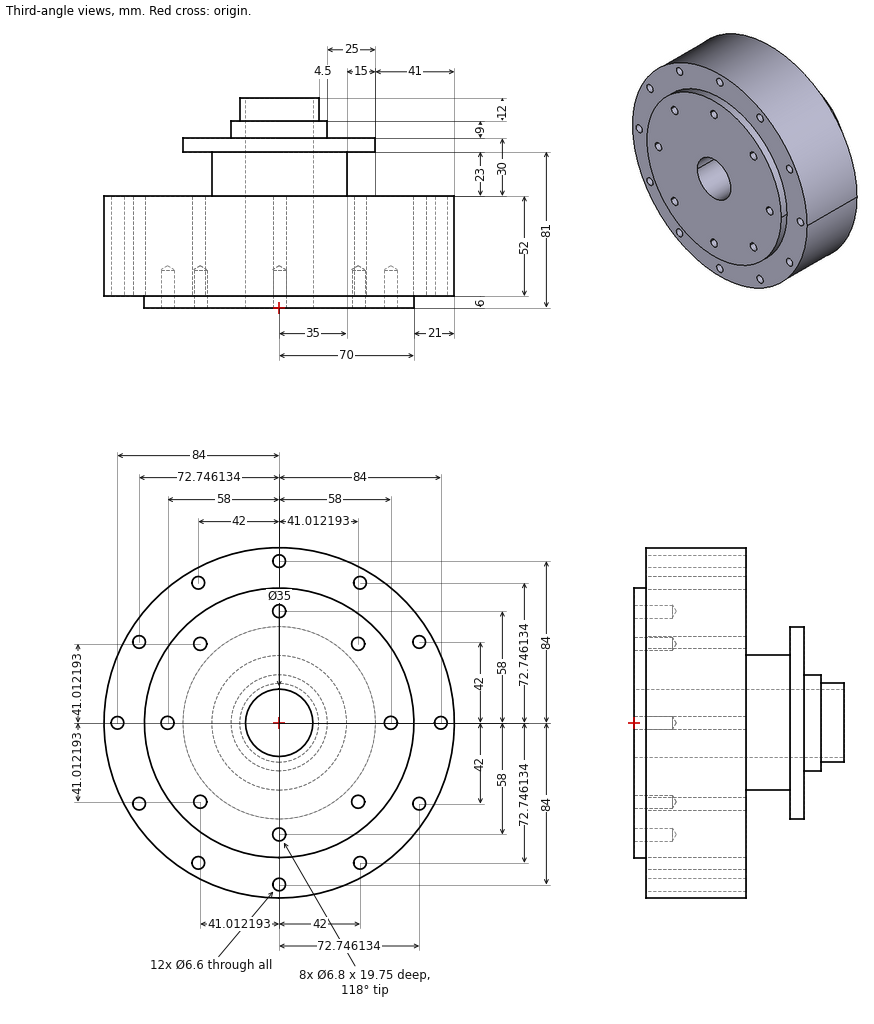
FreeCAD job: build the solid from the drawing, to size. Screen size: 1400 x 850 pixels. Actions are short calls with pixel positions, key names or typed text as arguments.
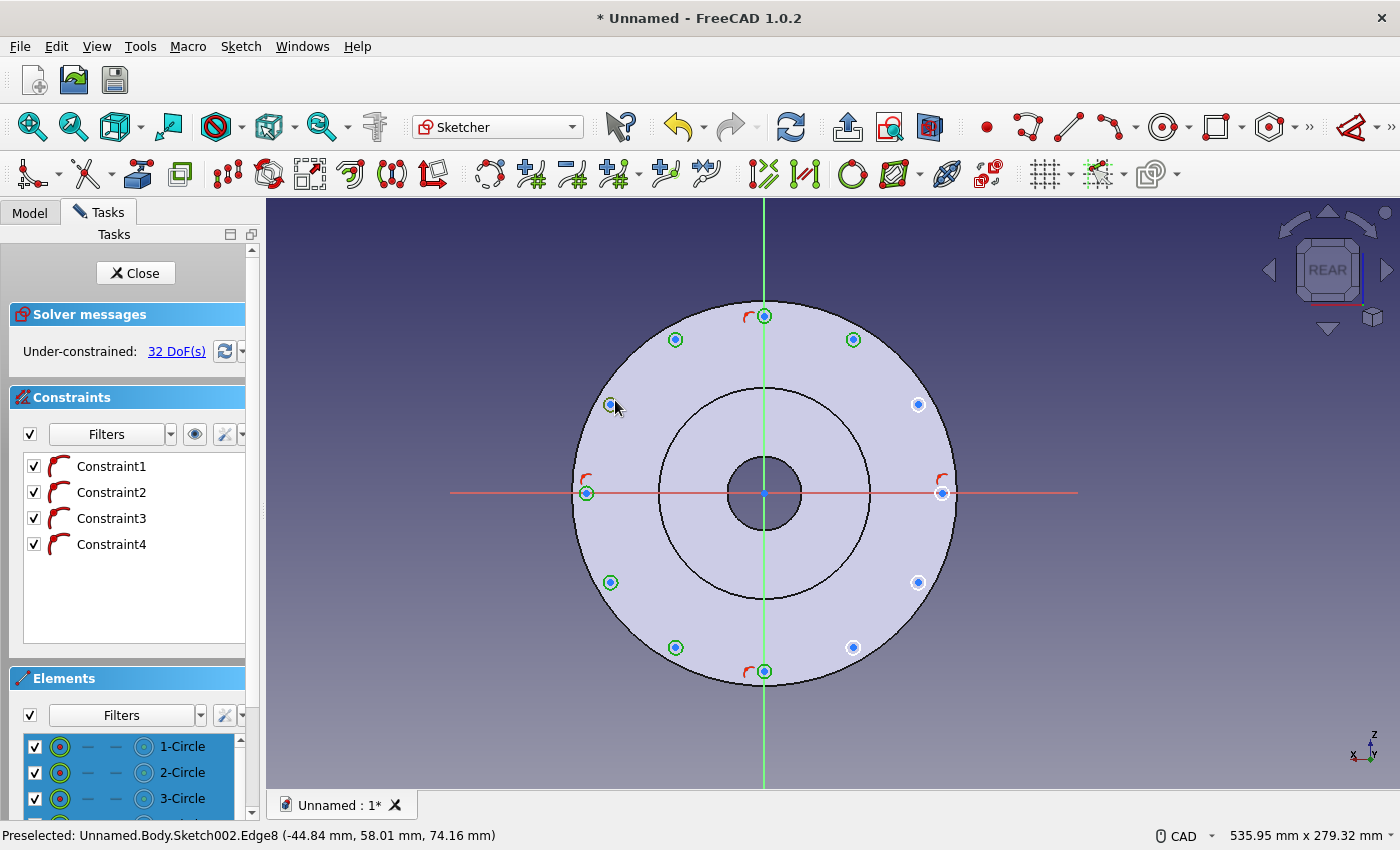
scroll(923, 400, up, 4)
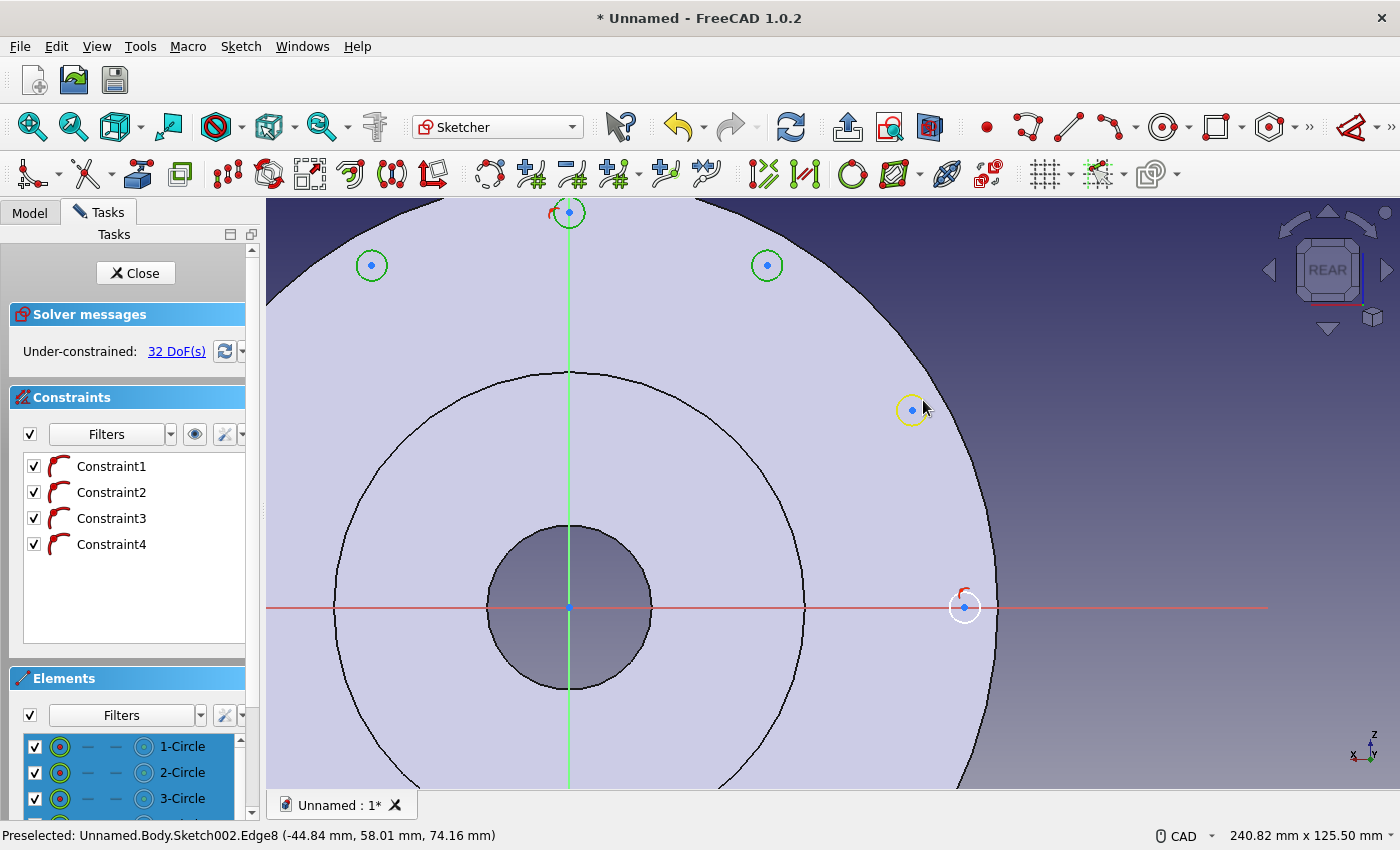
click(923, 400)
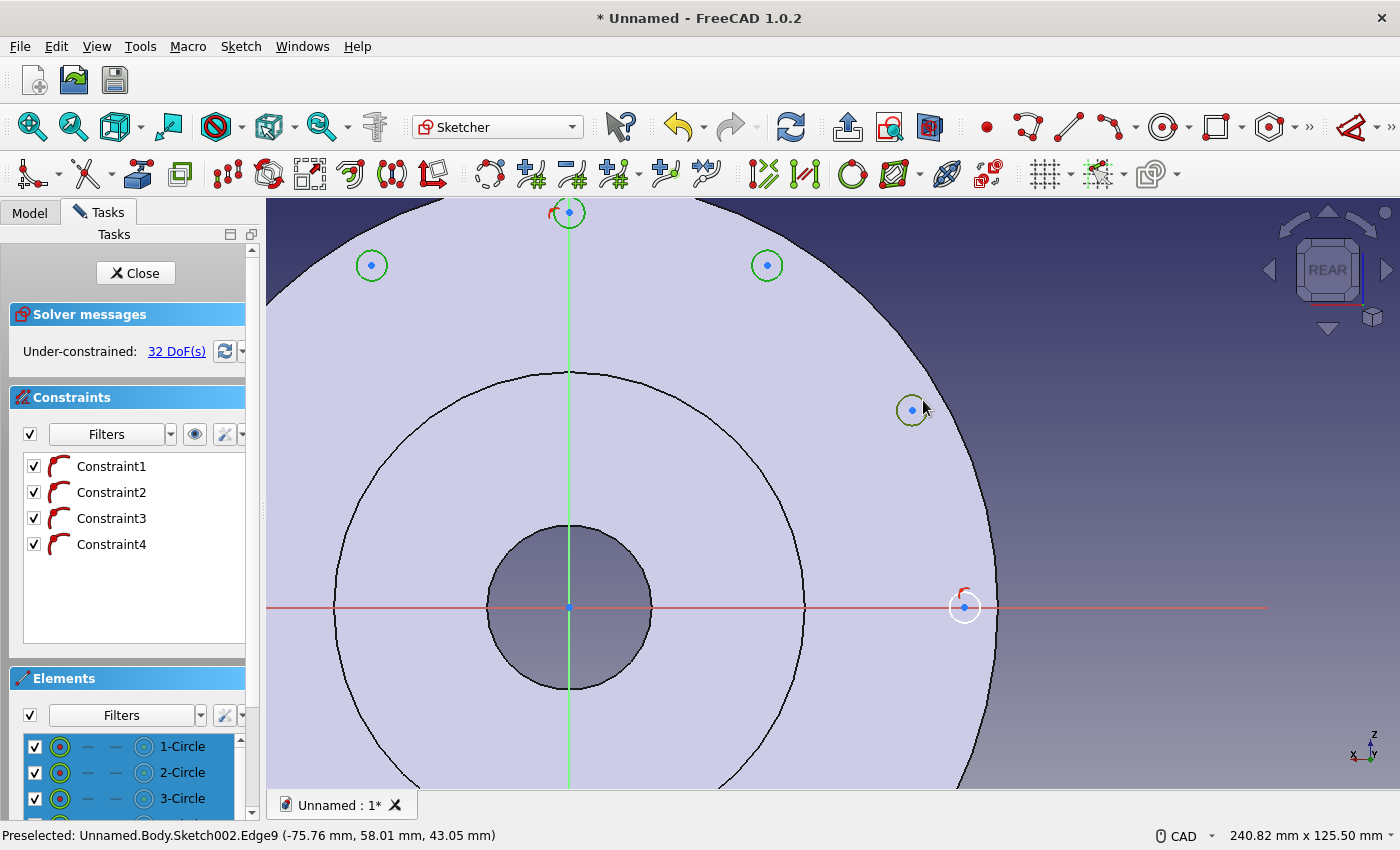
scroll(976, 597, up, 2)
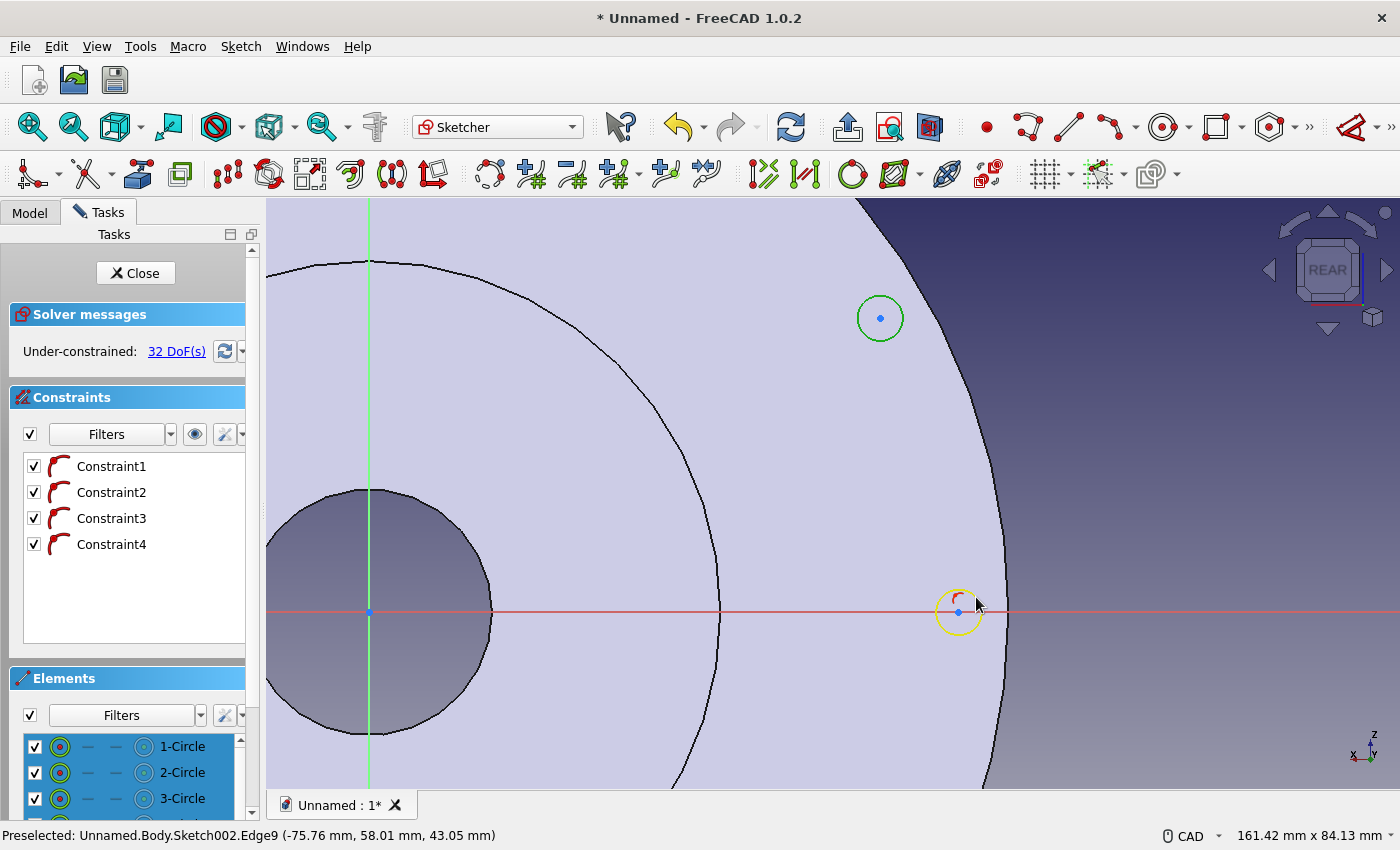
click(975, 596)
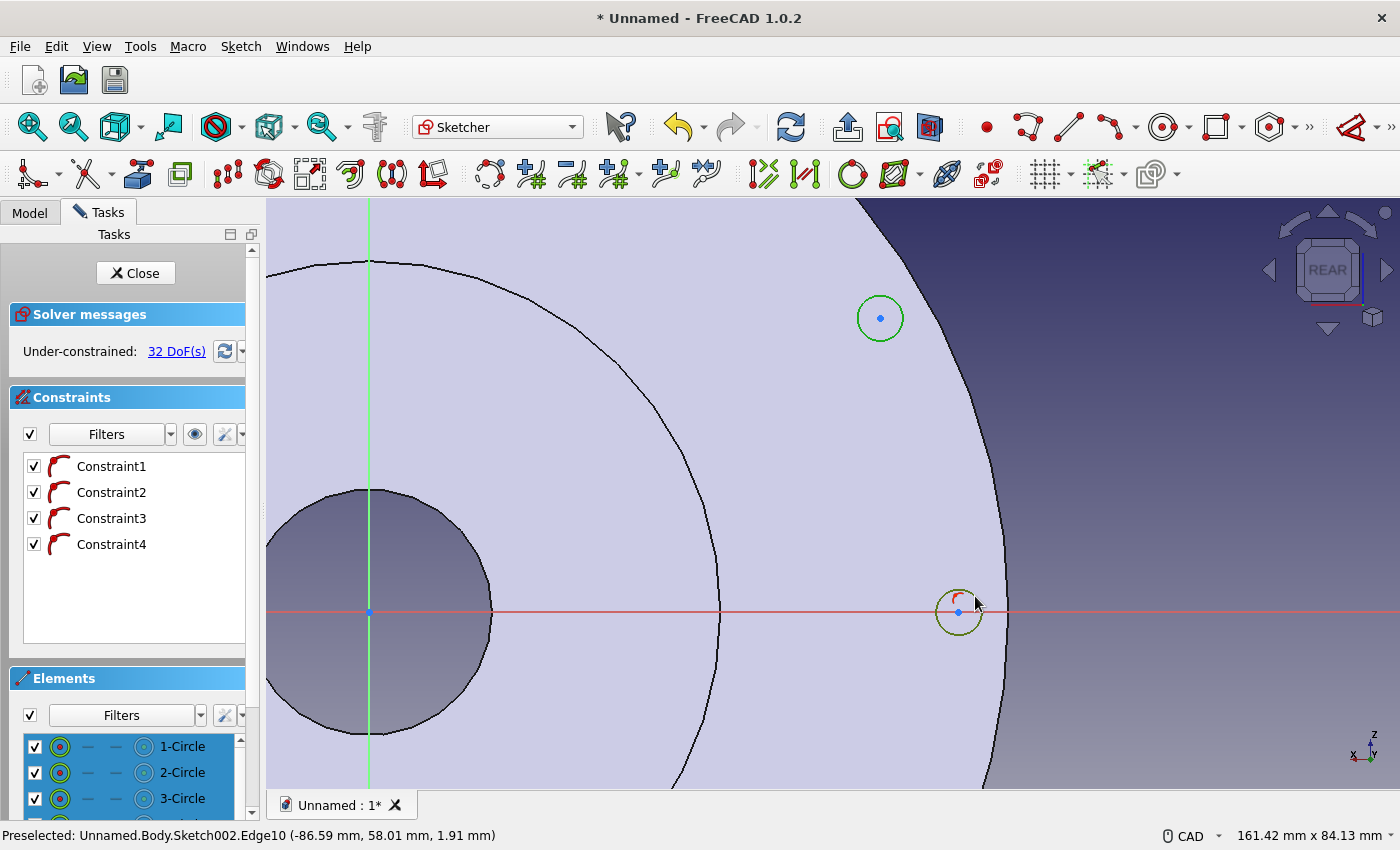
scroll(935, 442, down, 6)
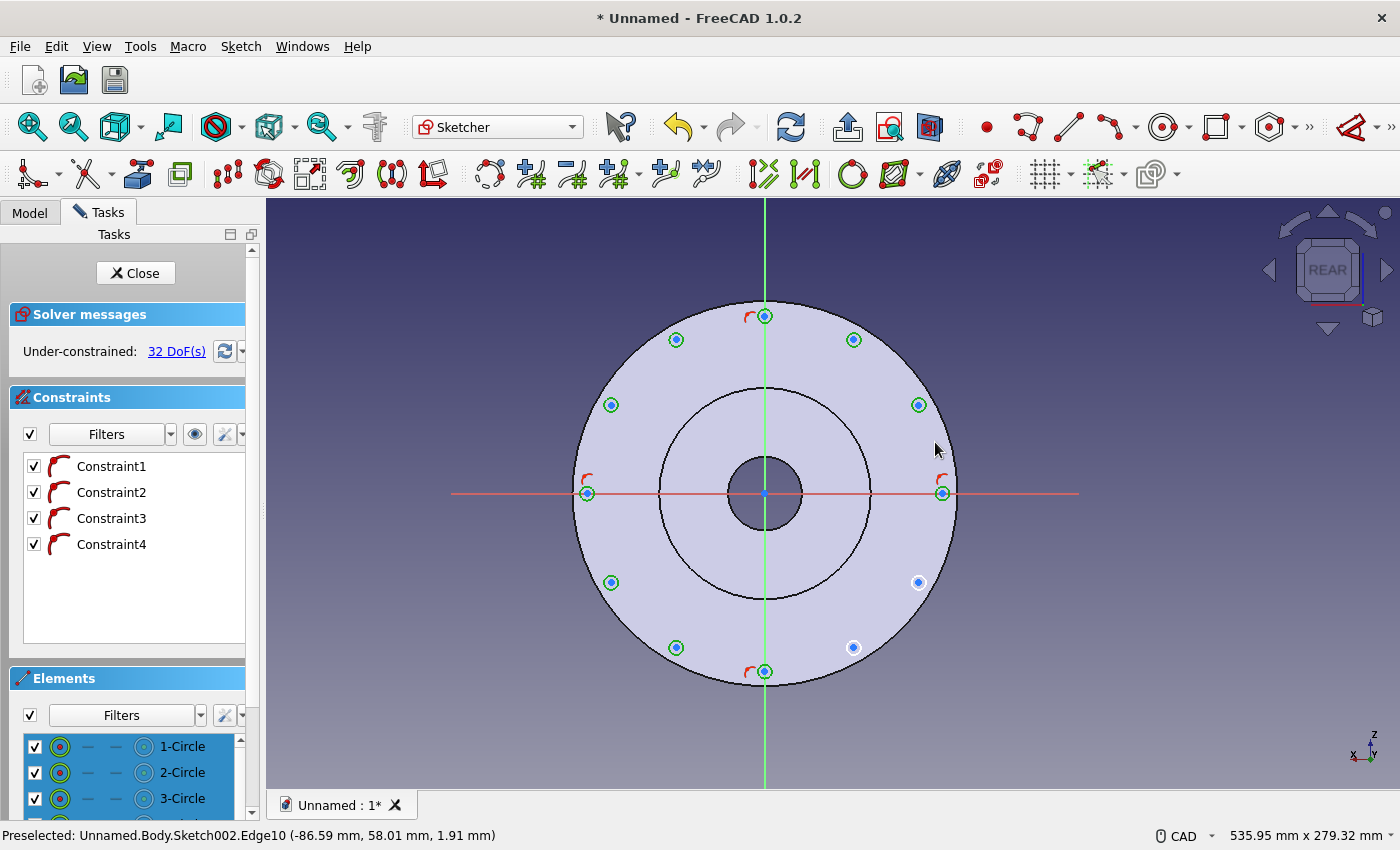
scroll(924, 578, up, 4)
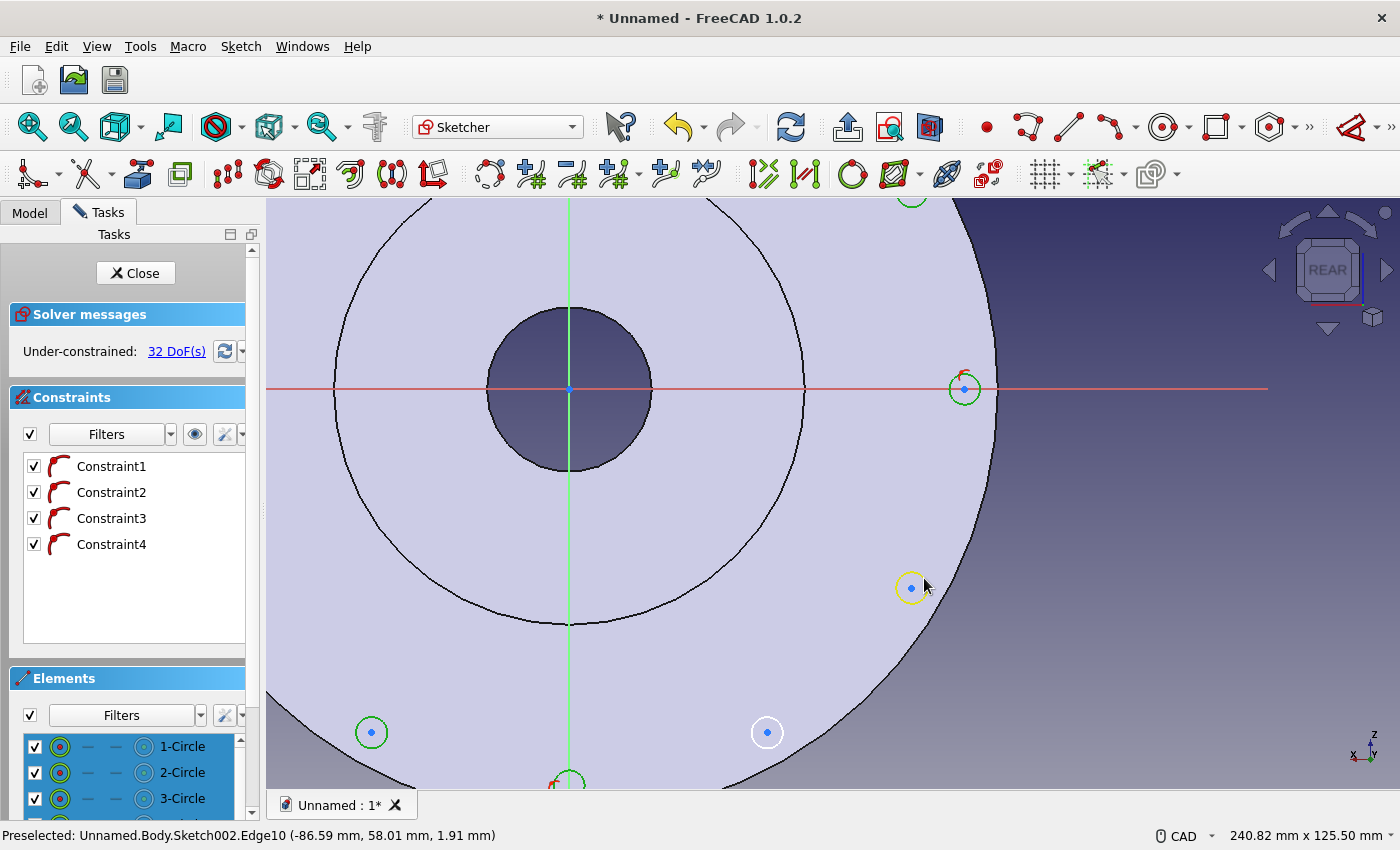
click(923, 577)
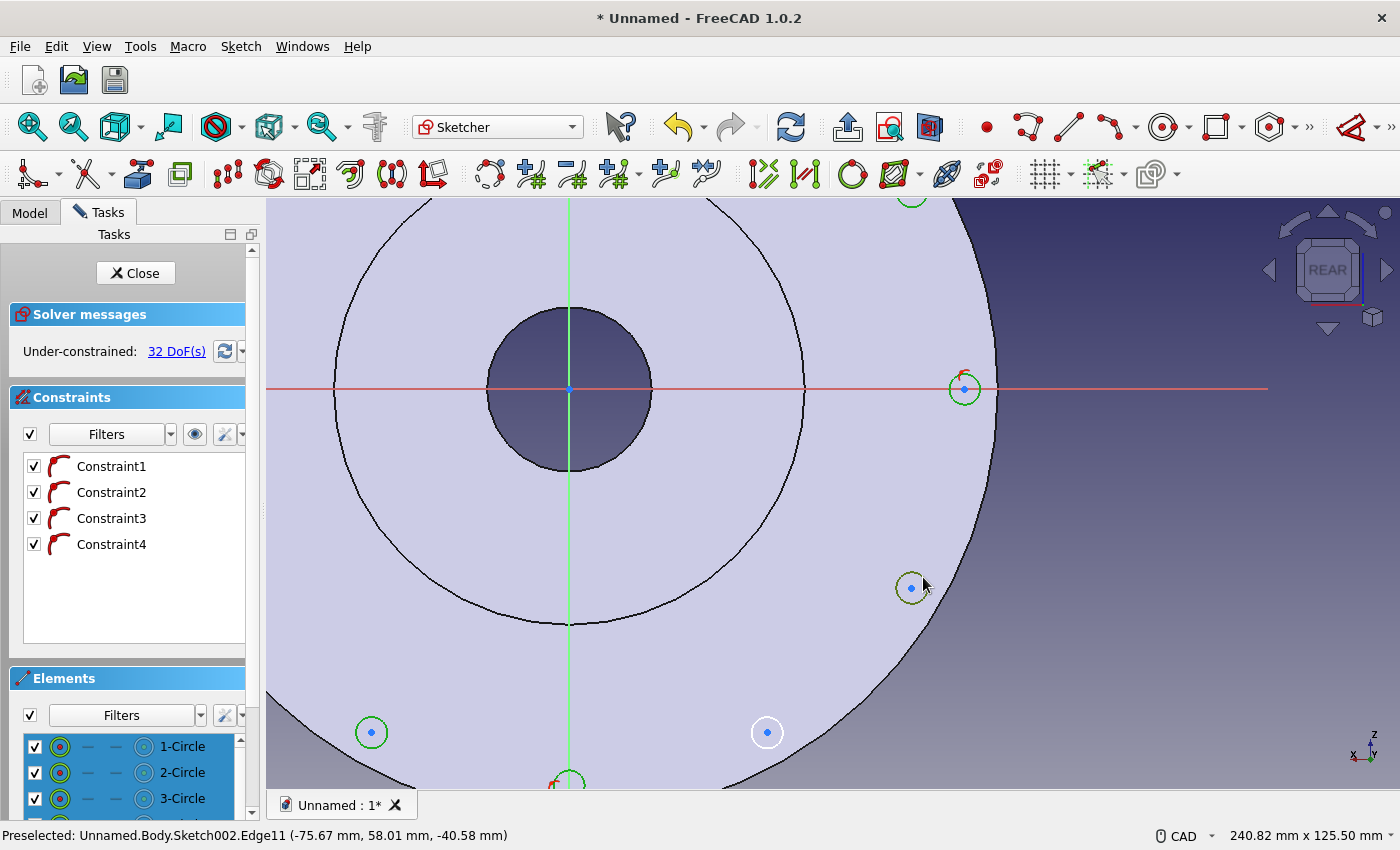
click(778, 722)